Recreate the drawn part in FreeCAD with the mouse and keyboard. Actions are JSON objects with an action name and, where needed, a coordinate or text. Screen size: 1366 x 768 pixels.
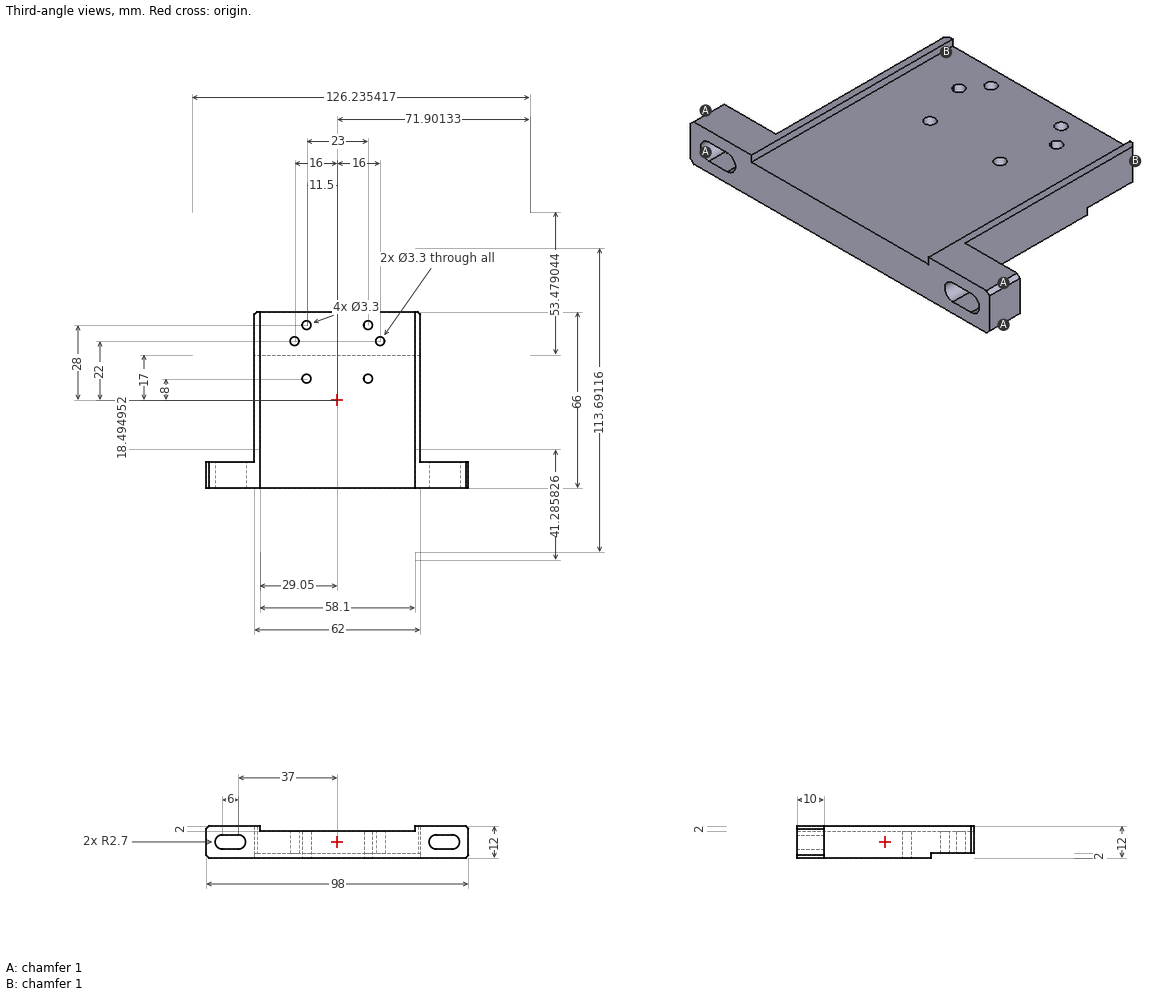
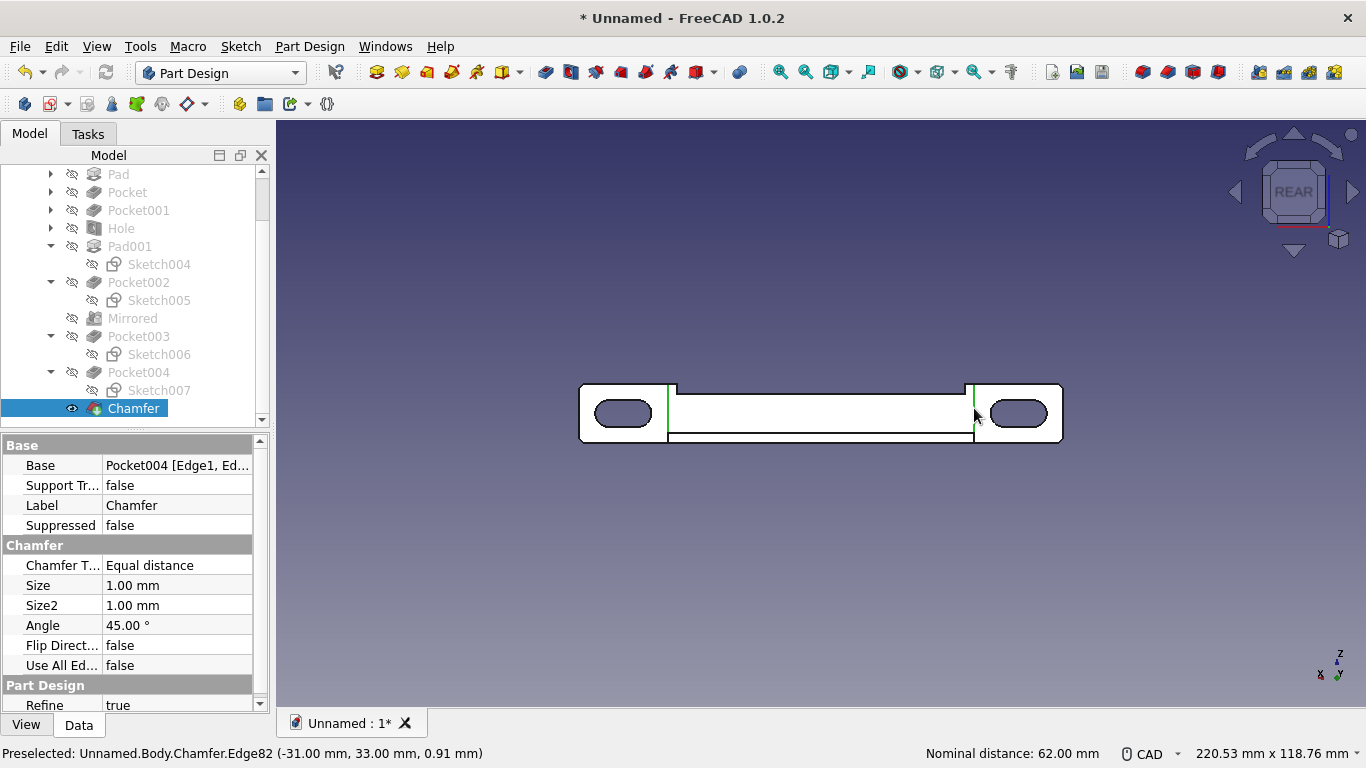
{"action": "left_click", "coordinate": [1168, 72]}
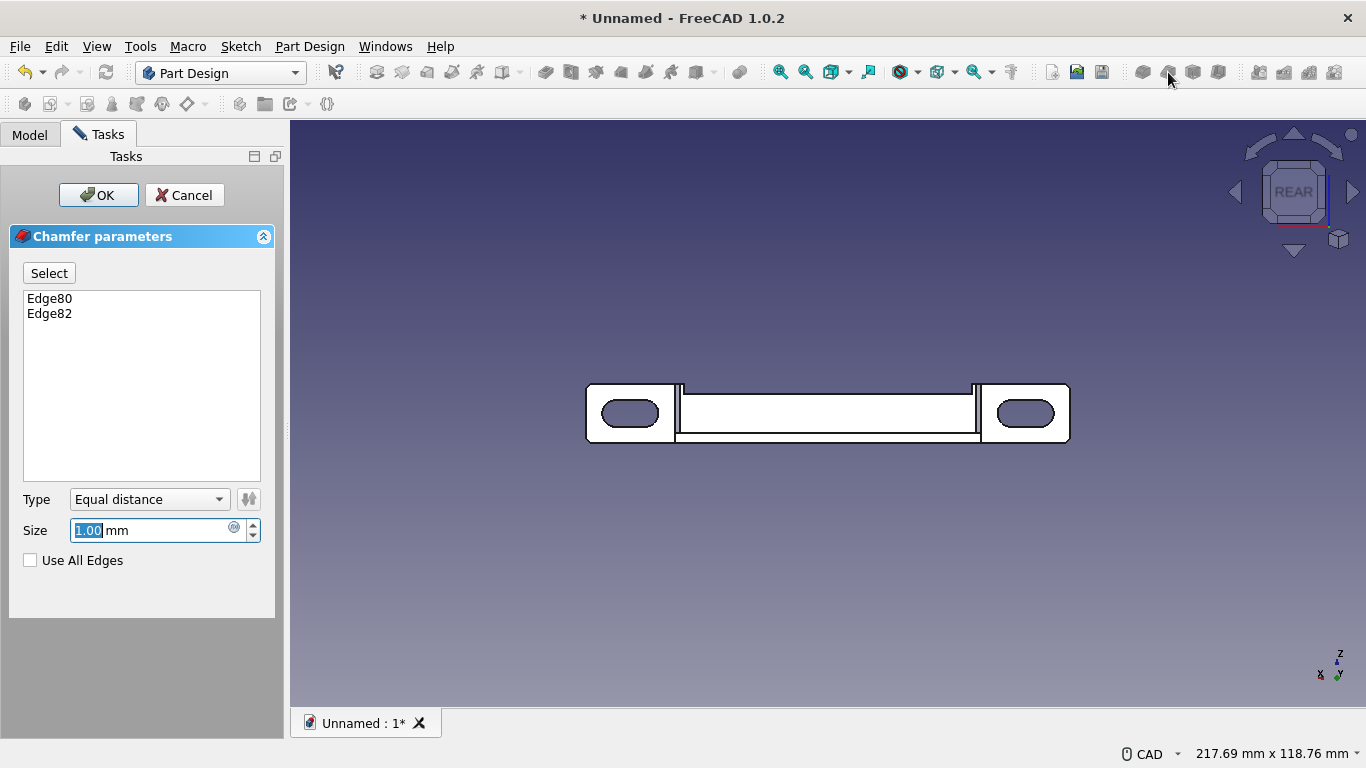
{"action": "type", "text": "1"}
{"action": "key", "text": "Tab"}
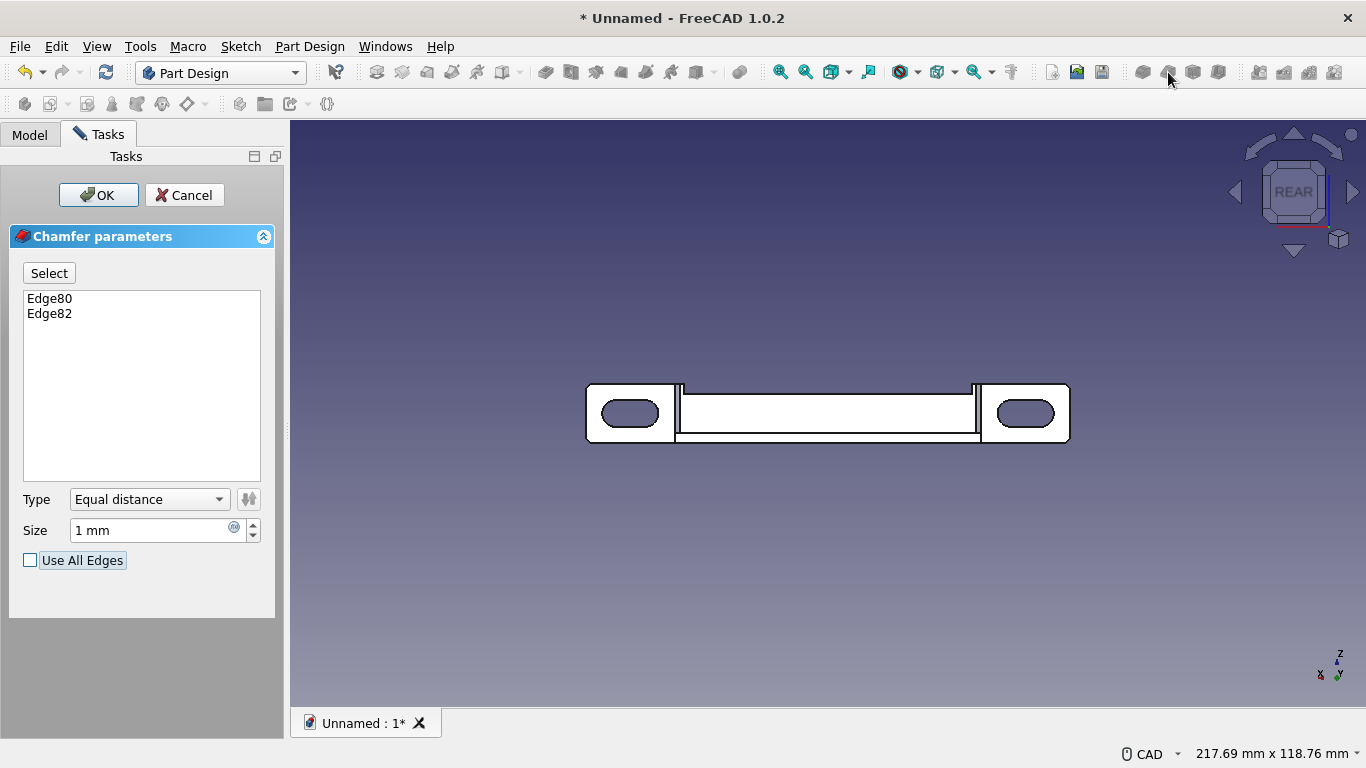
{"action": "left_click", "coordinate": [99, 195]}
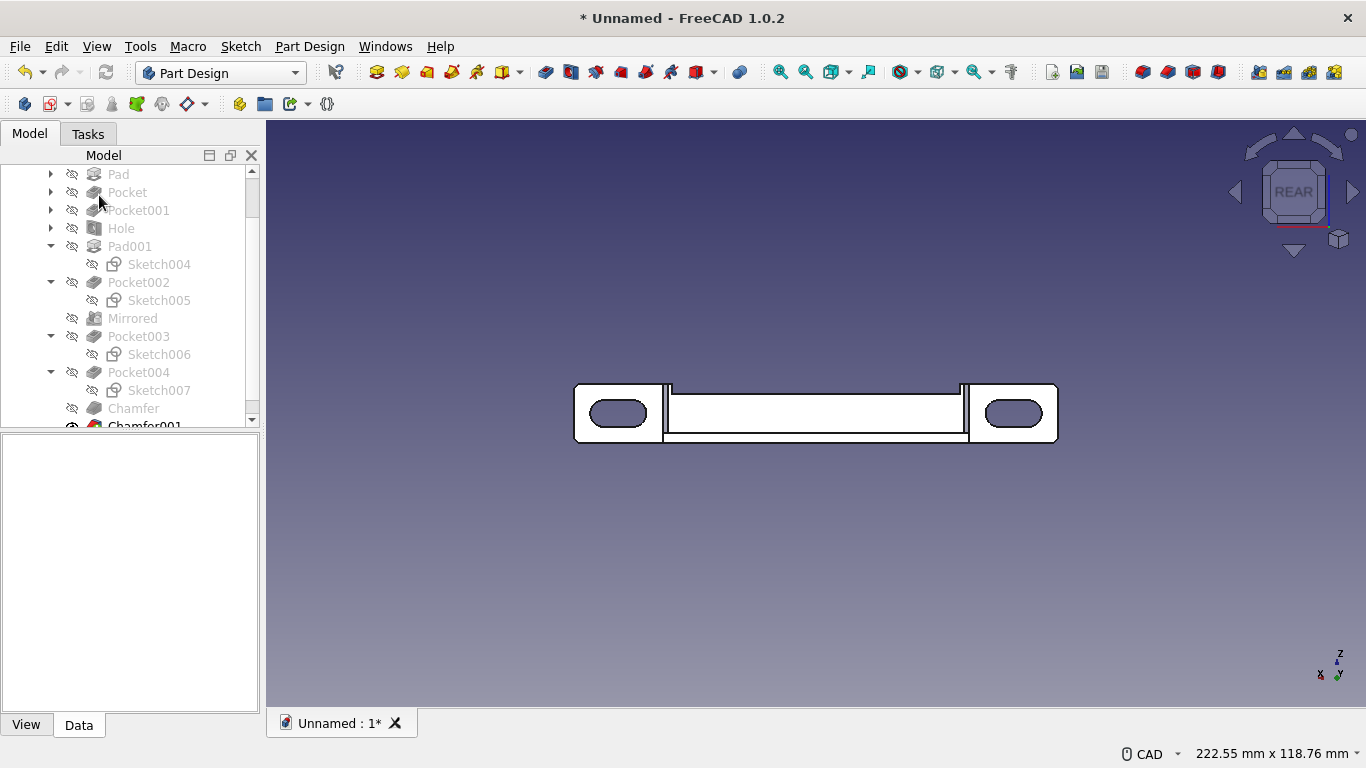
{"action": "key", "text": "0"}